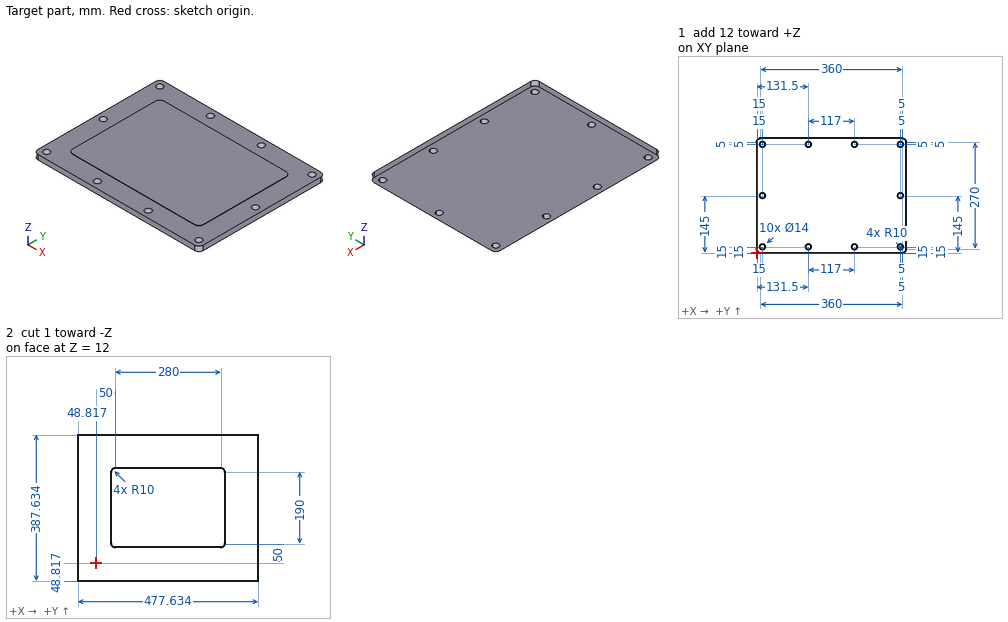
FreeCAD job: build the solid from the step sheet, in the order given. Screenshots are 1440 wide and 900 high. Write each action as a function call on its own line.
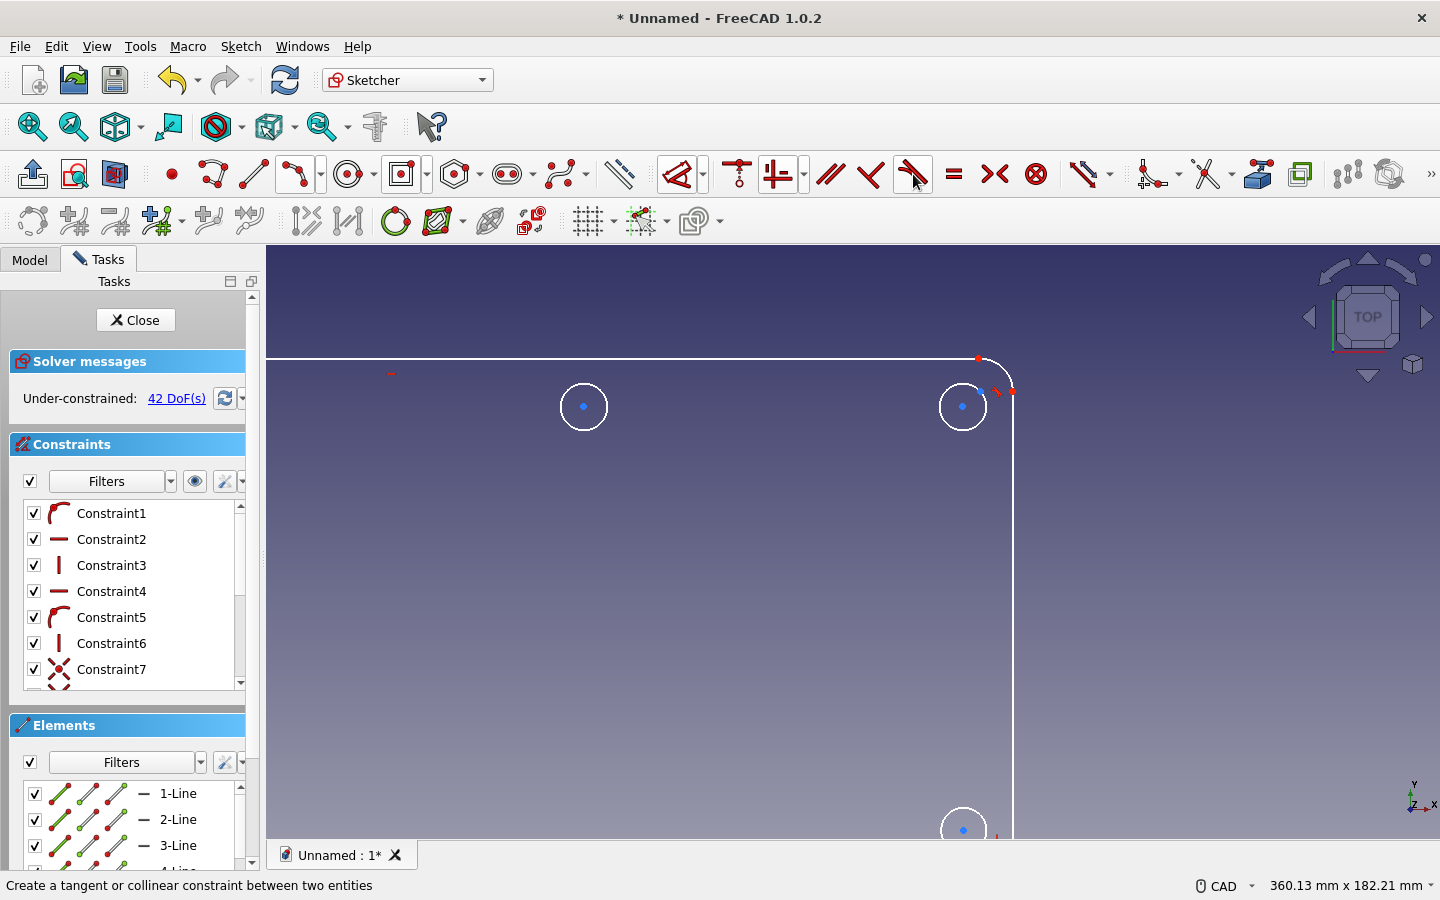
click(627, 359)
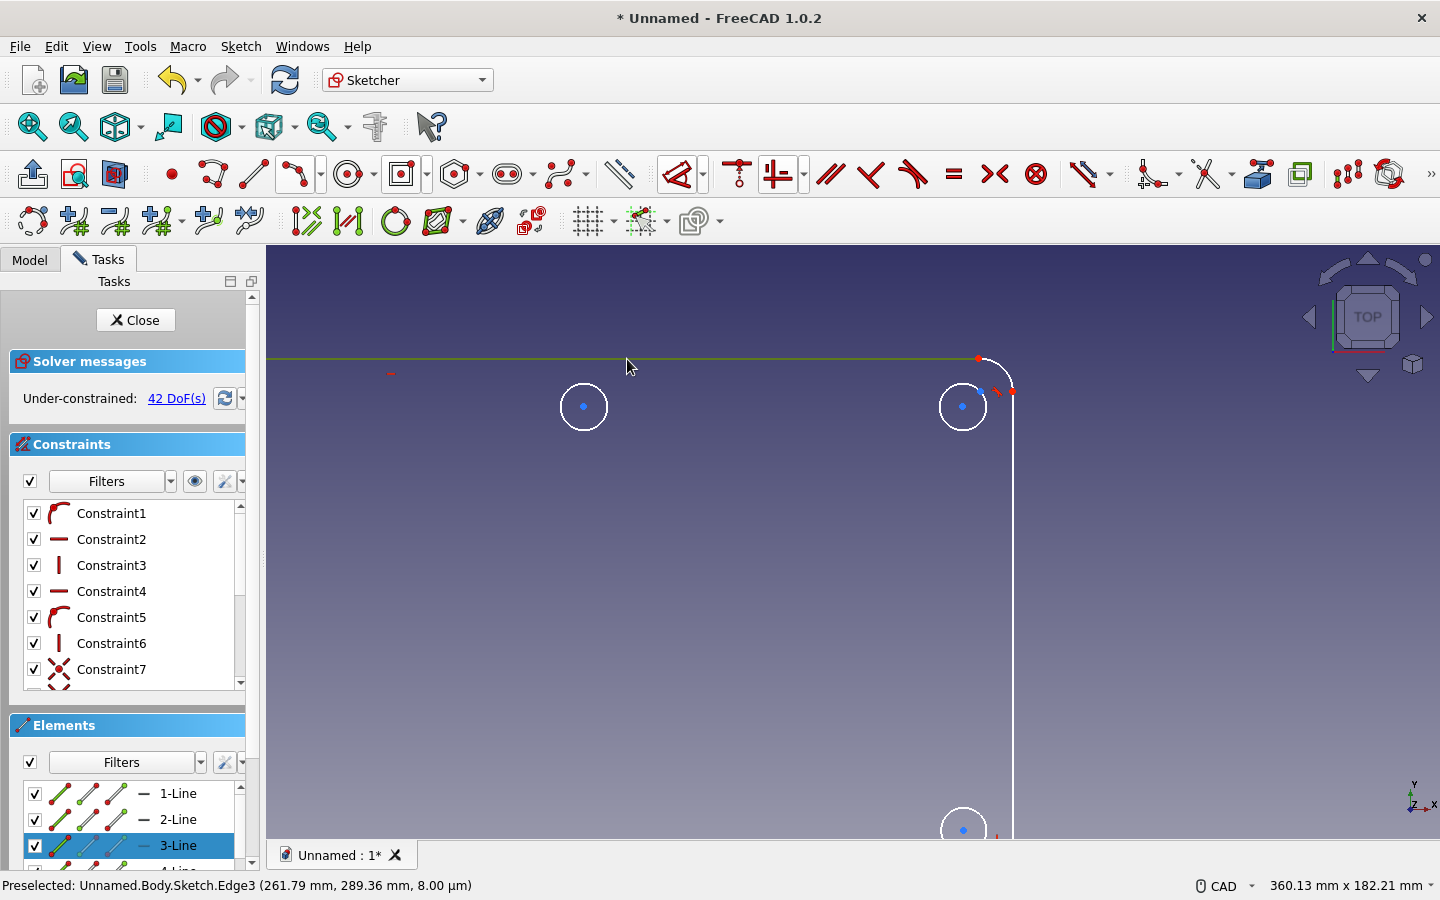
click(1009, 376)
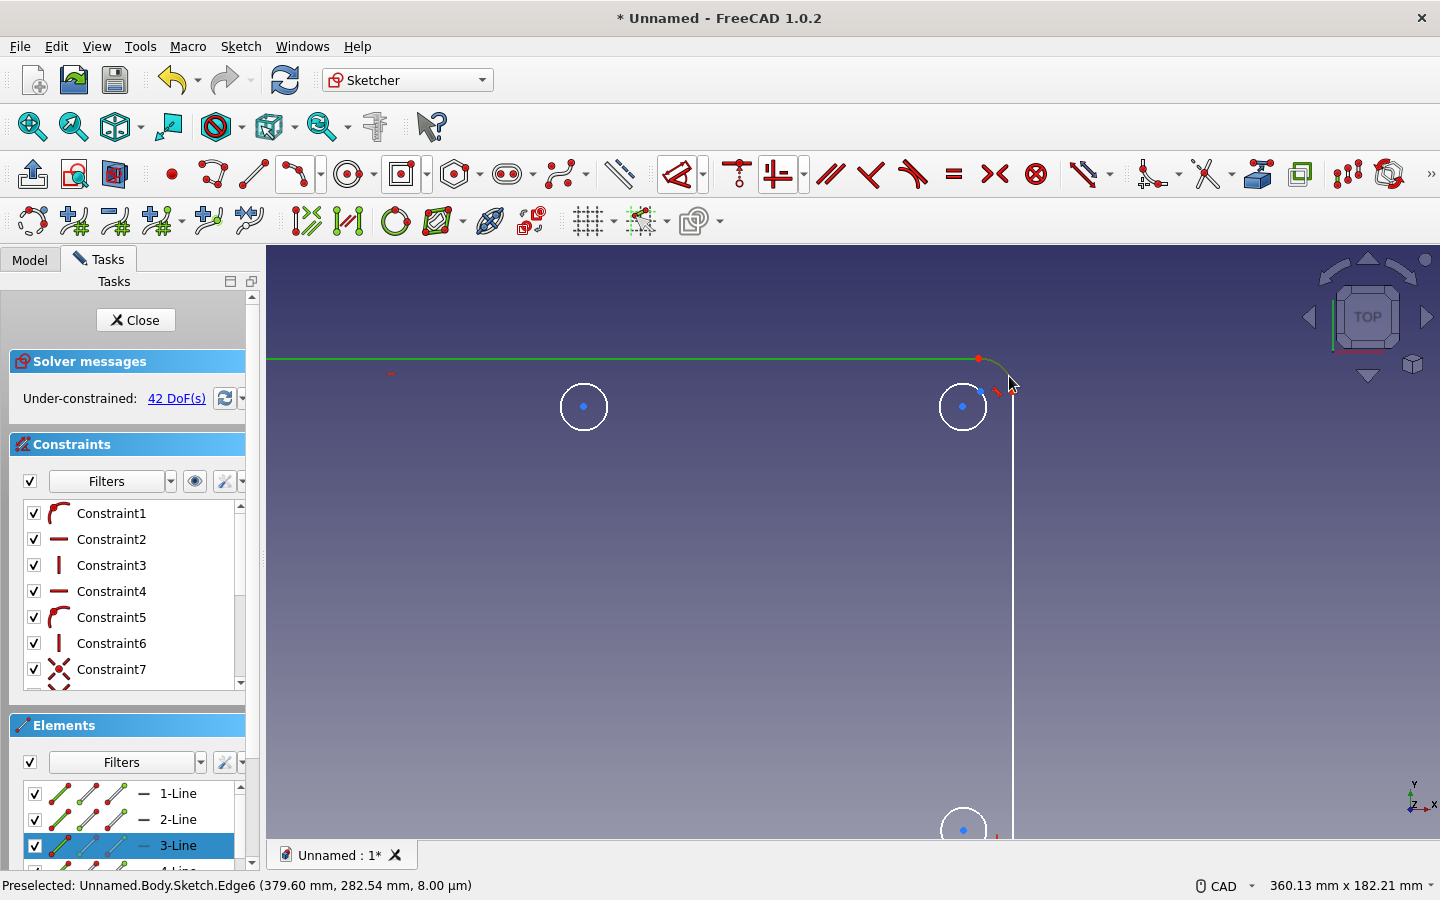
click(913, 174)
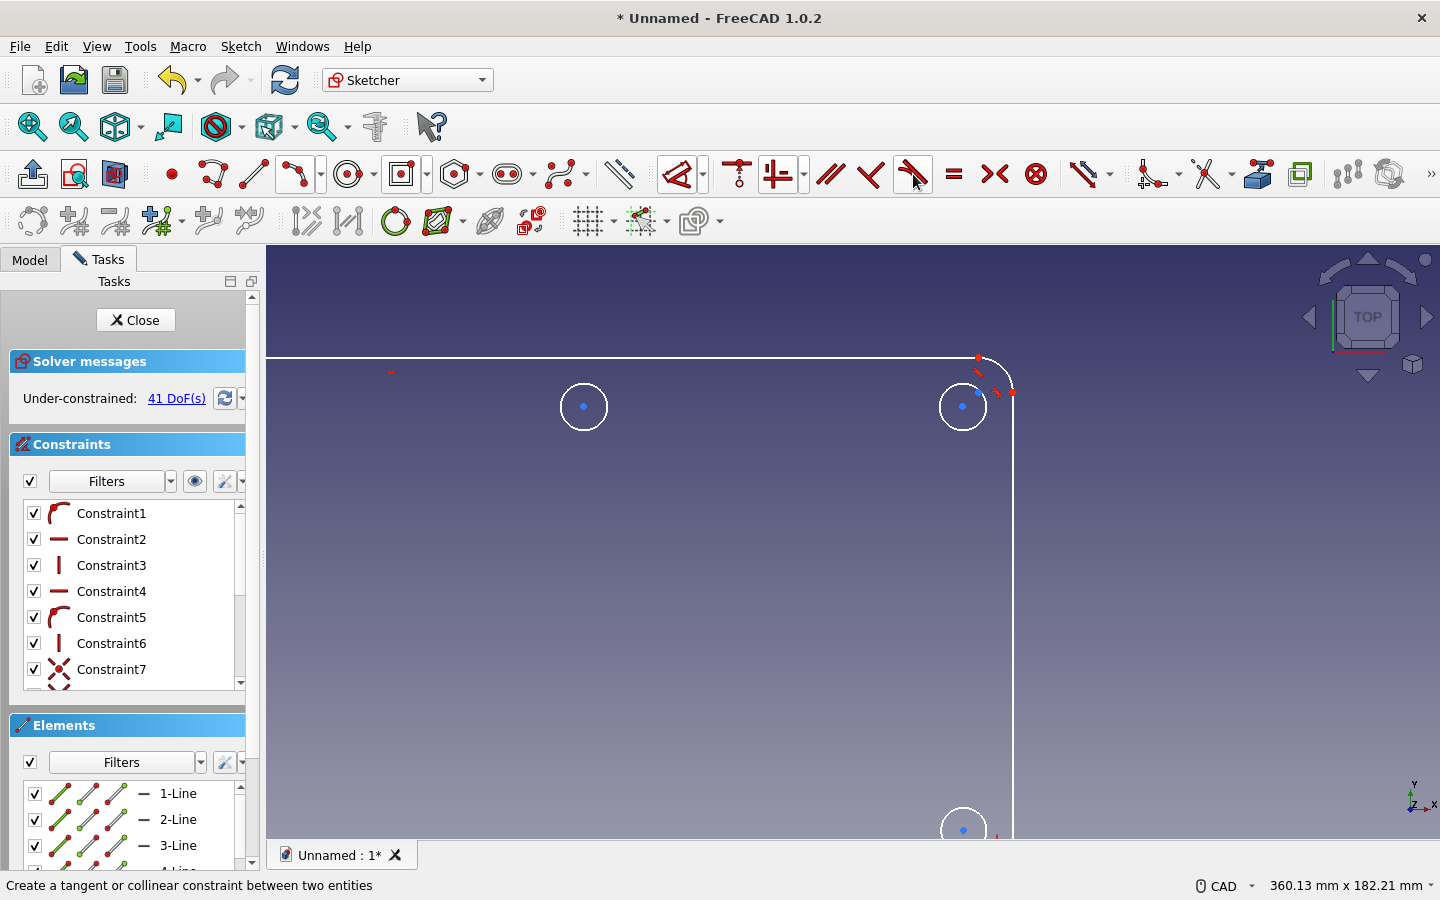
click(627, 358)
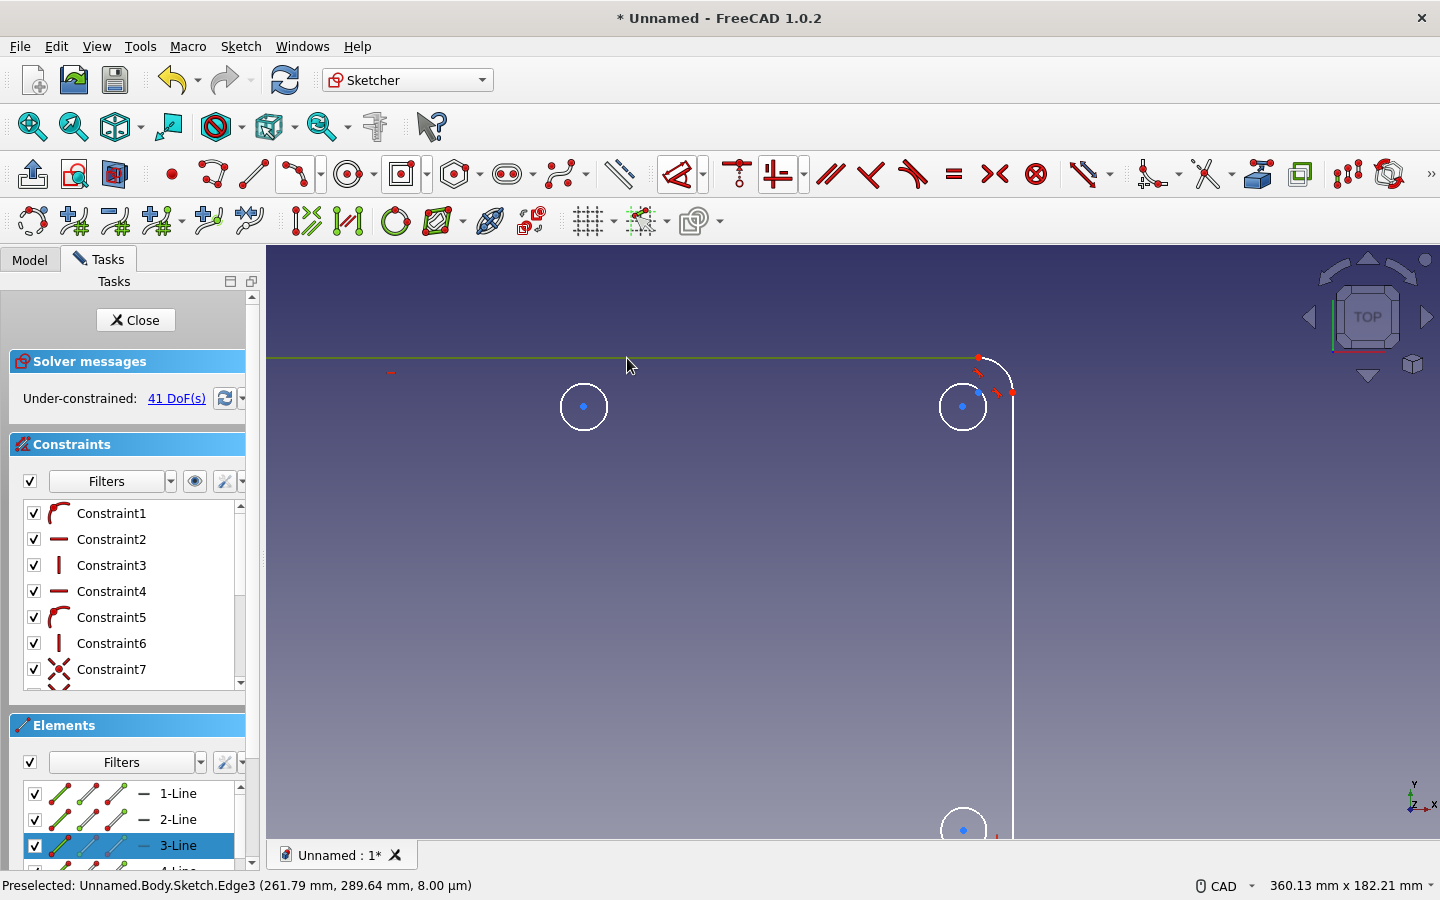
scroll(1012, 375, down, 5)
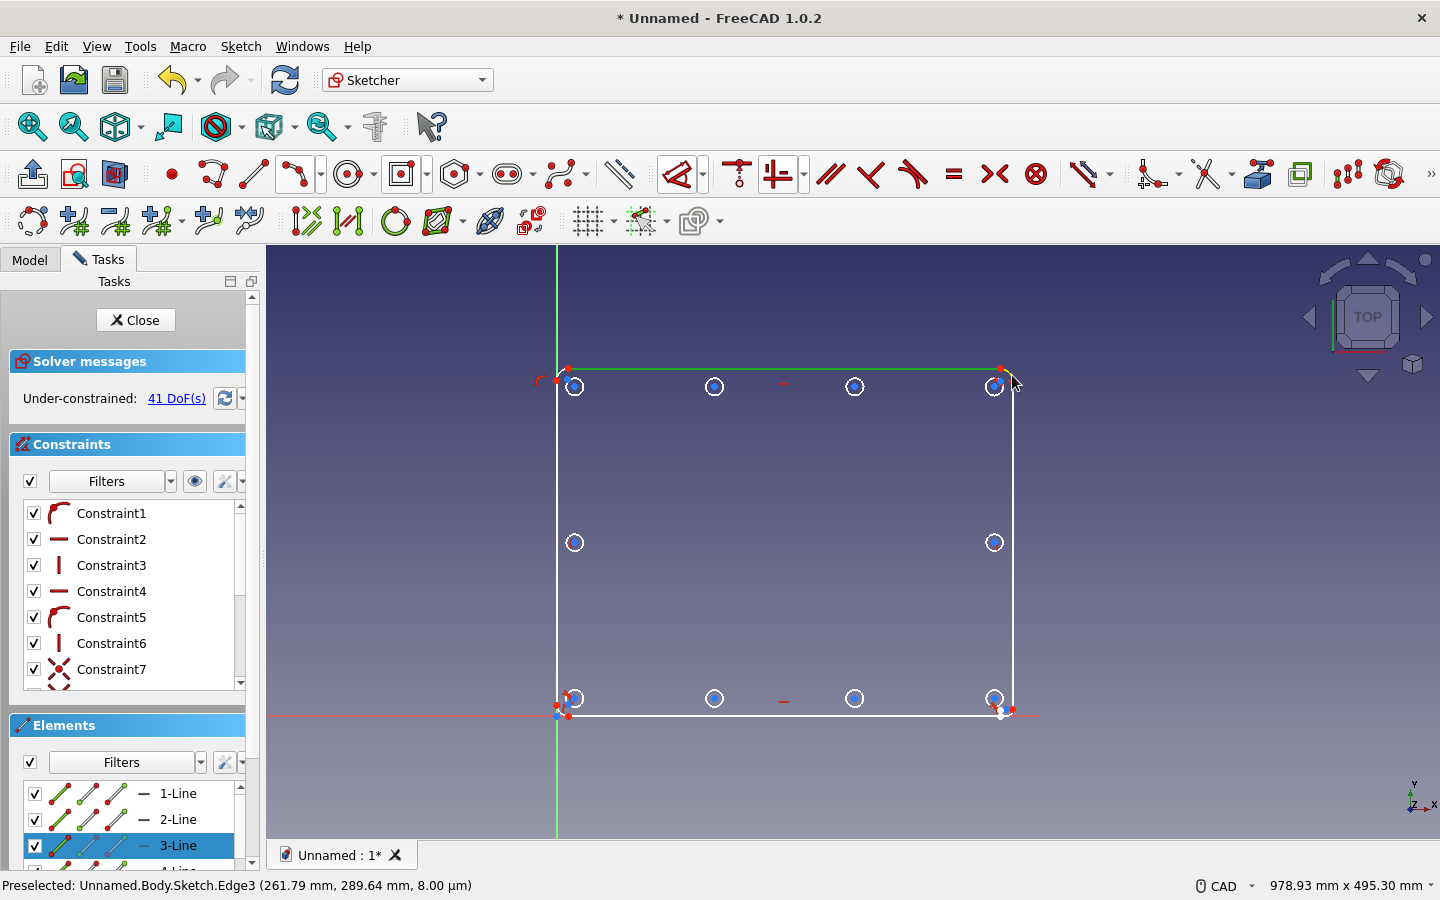
scroll(563, 370, up, 5)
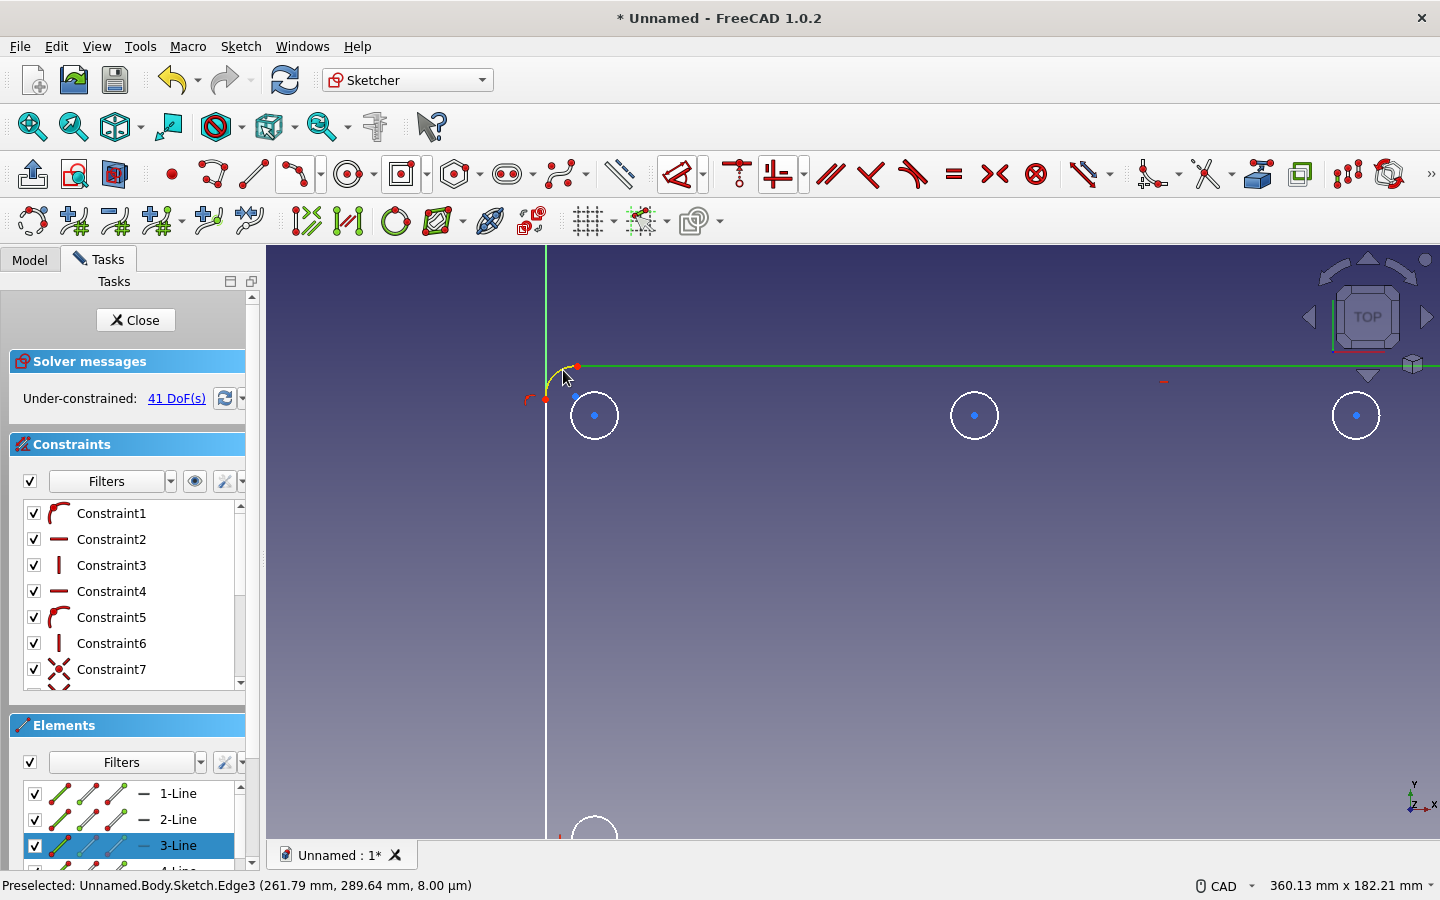
click(562, 369)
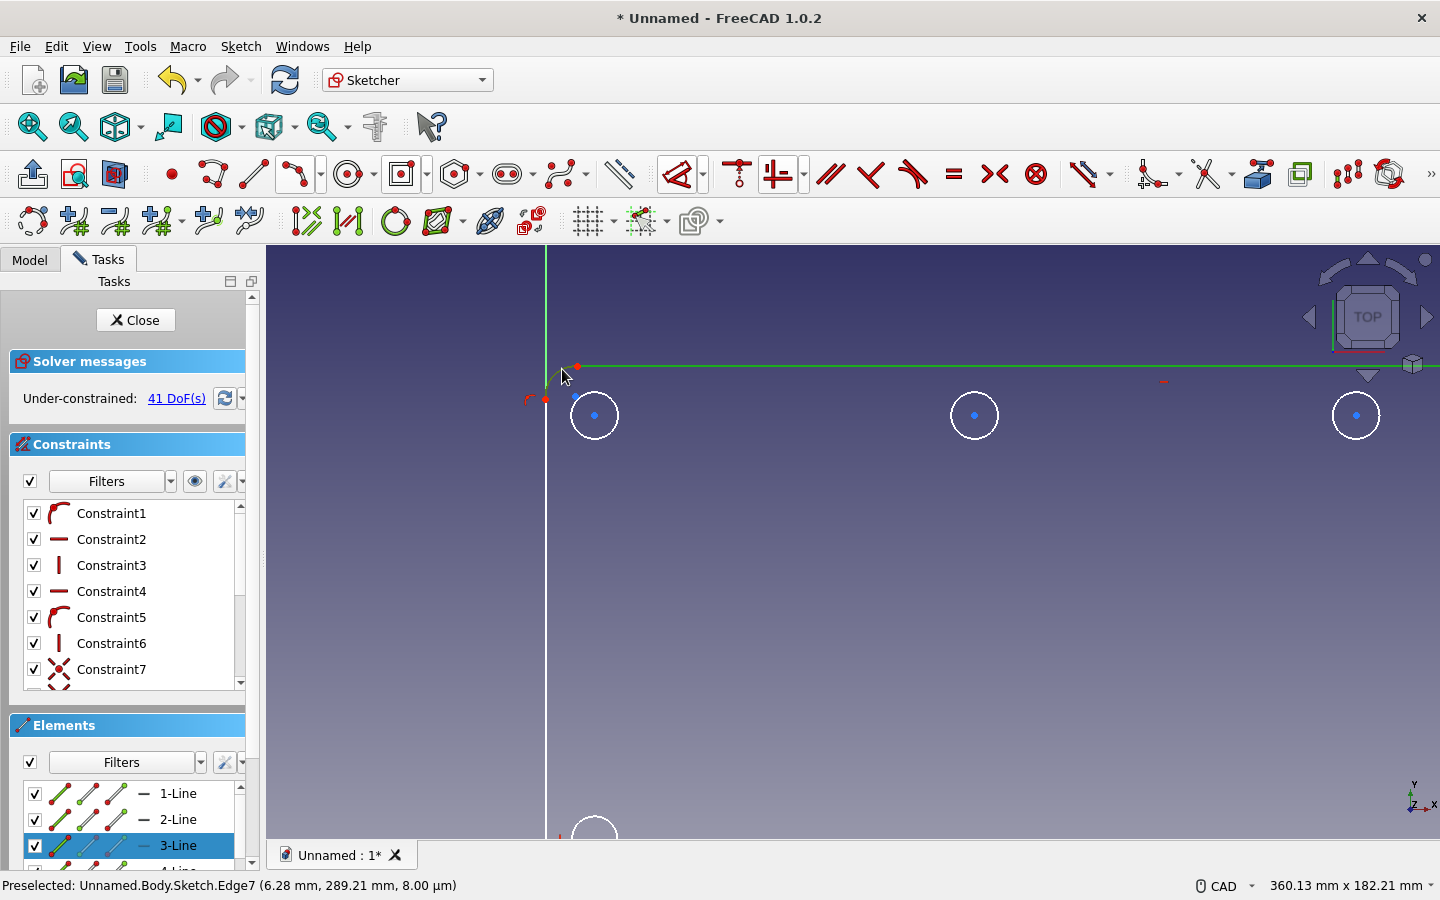
click(913, 174)